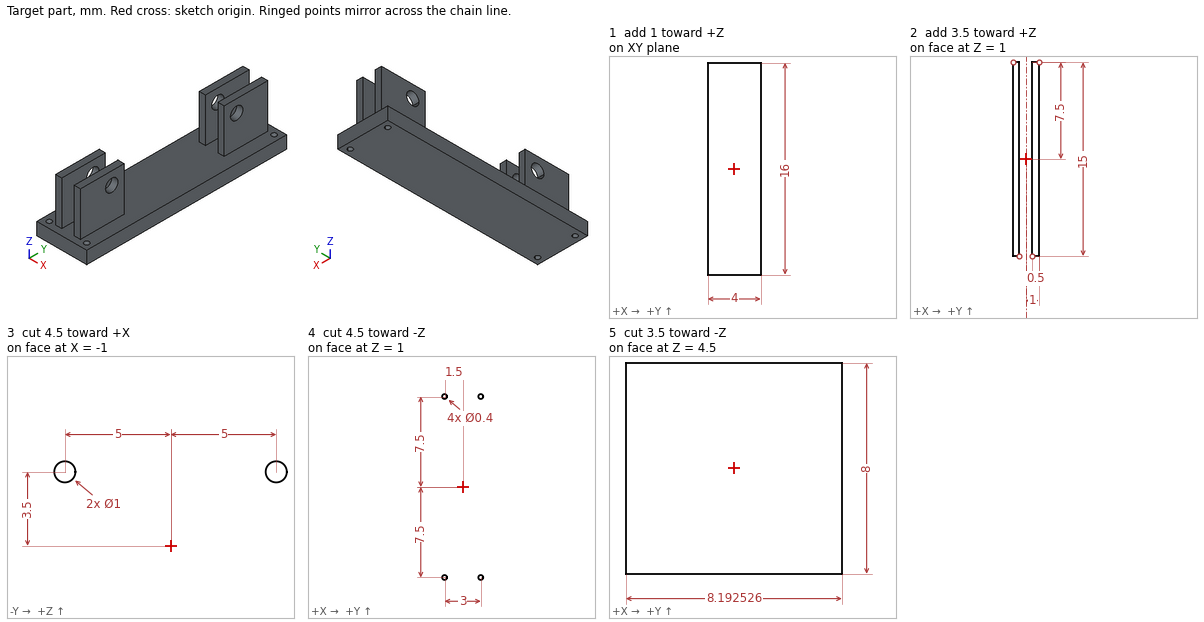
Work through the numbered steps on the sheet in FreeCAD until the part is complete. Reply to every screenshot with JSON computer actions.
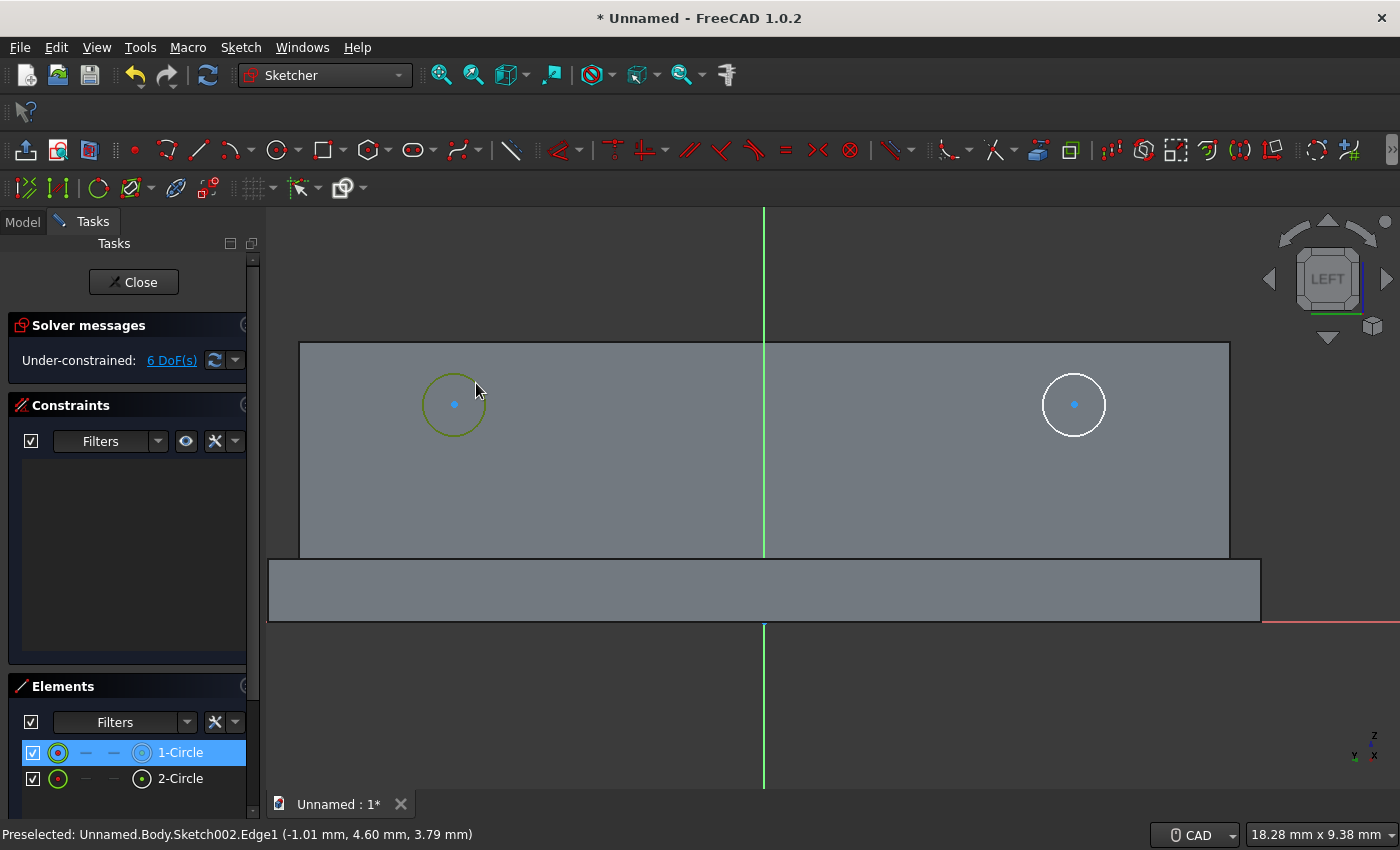
{"action": "left_click", "coordinate": [1096, 383]}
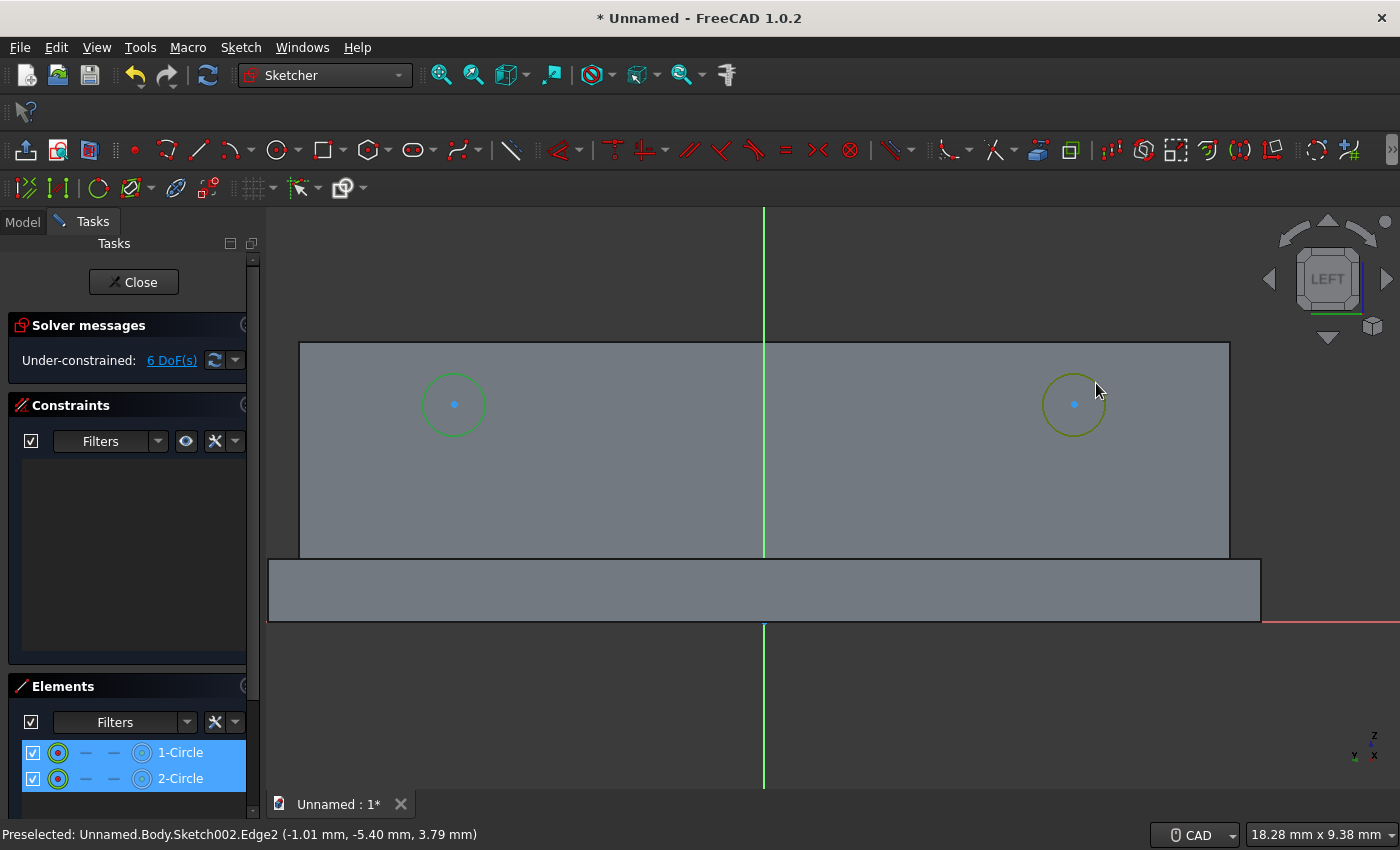
{"action": "key", "text": "e"}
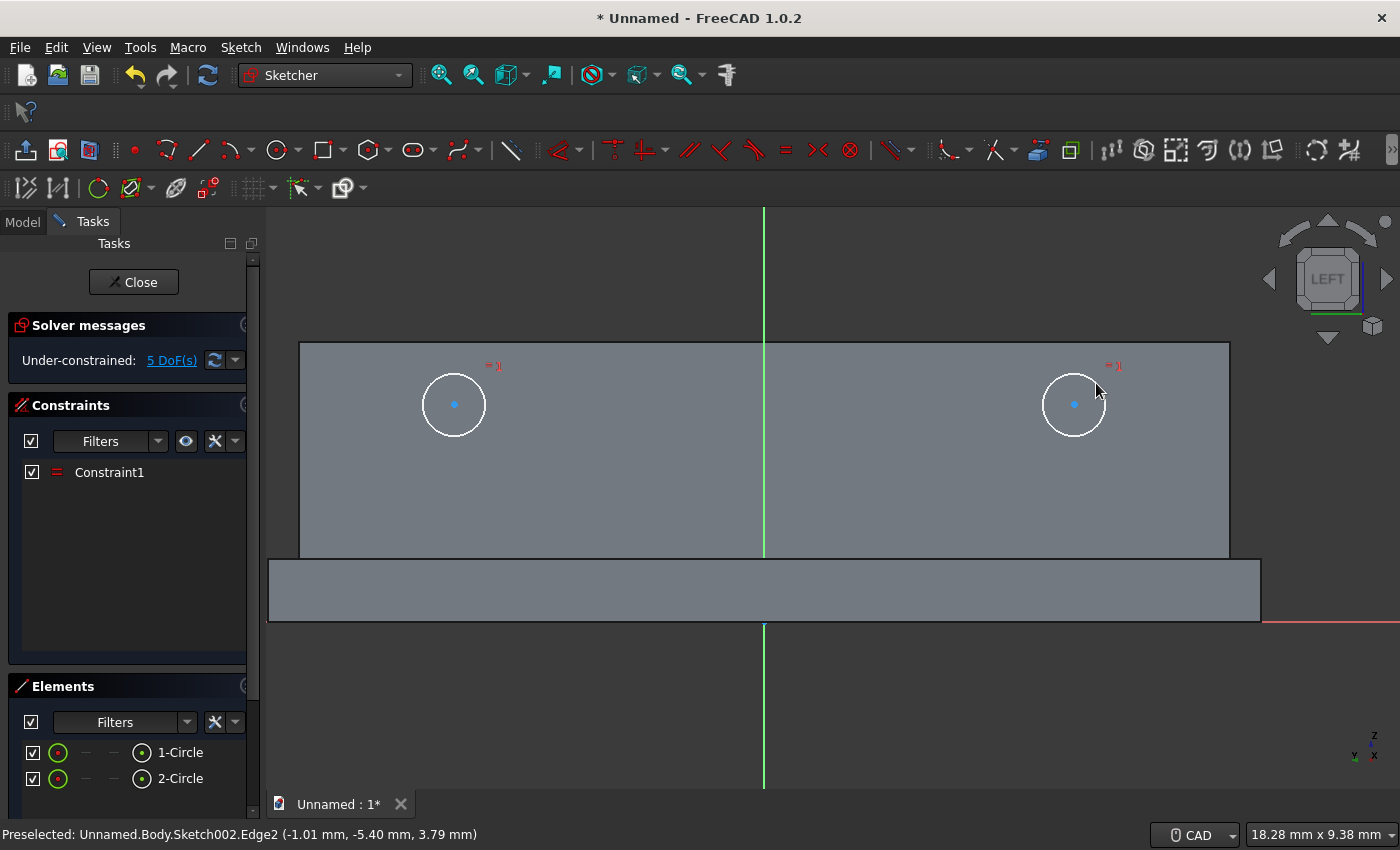
{"action": "left_click", "coordinate": [454, 405]}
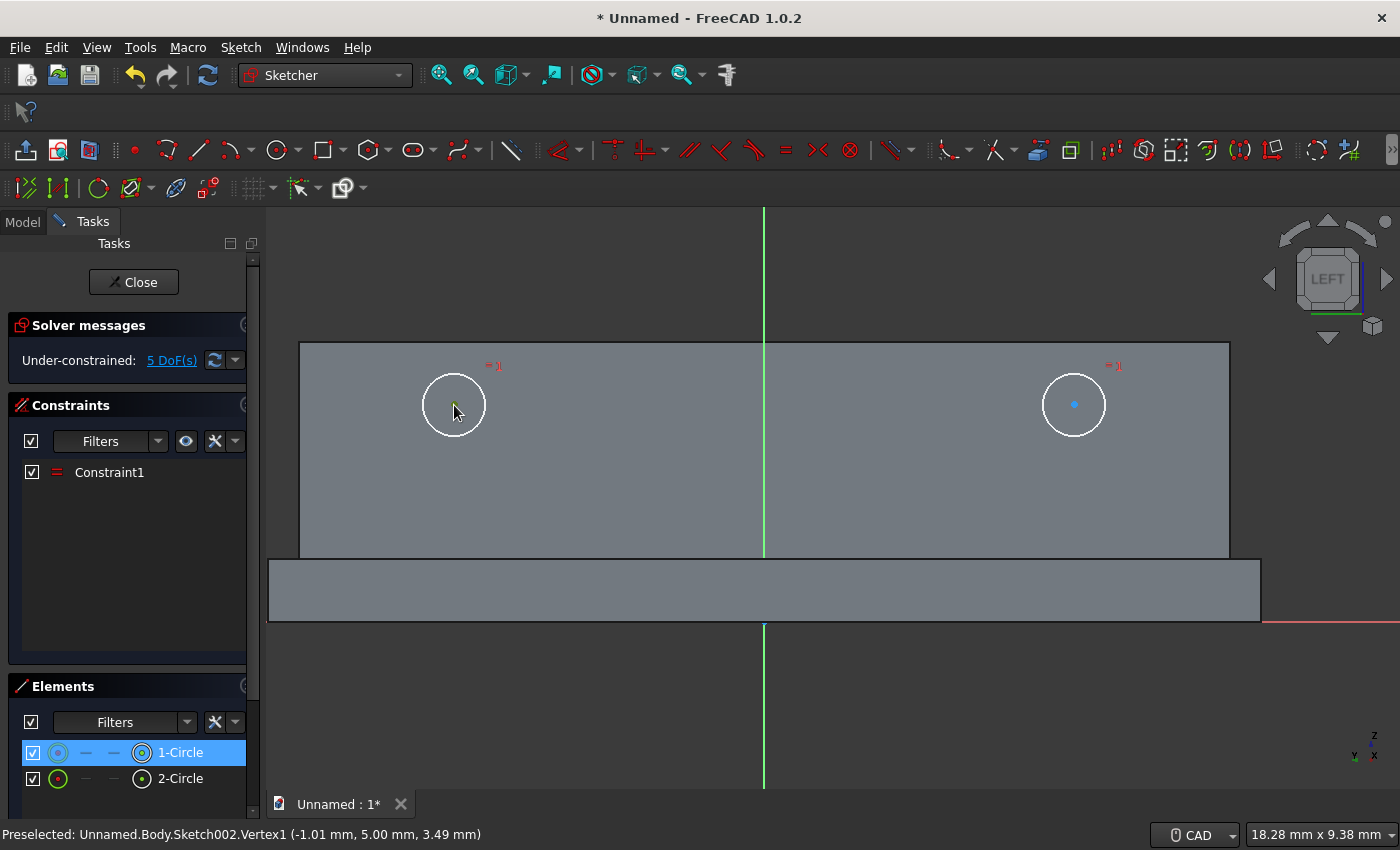
{"action": "left_click", "coordinate": [1074, 405]}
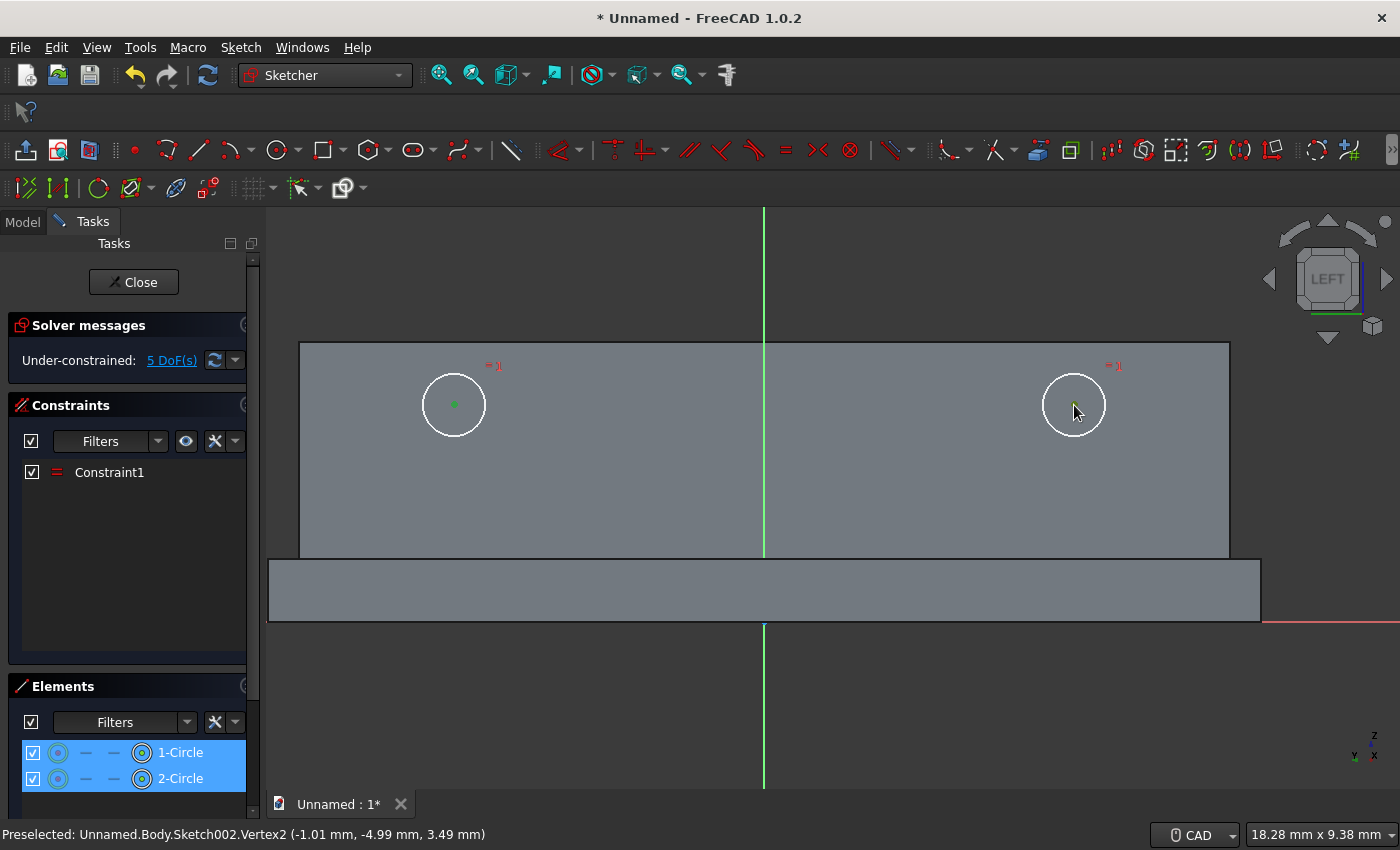
{"action": "key", "text": "h"}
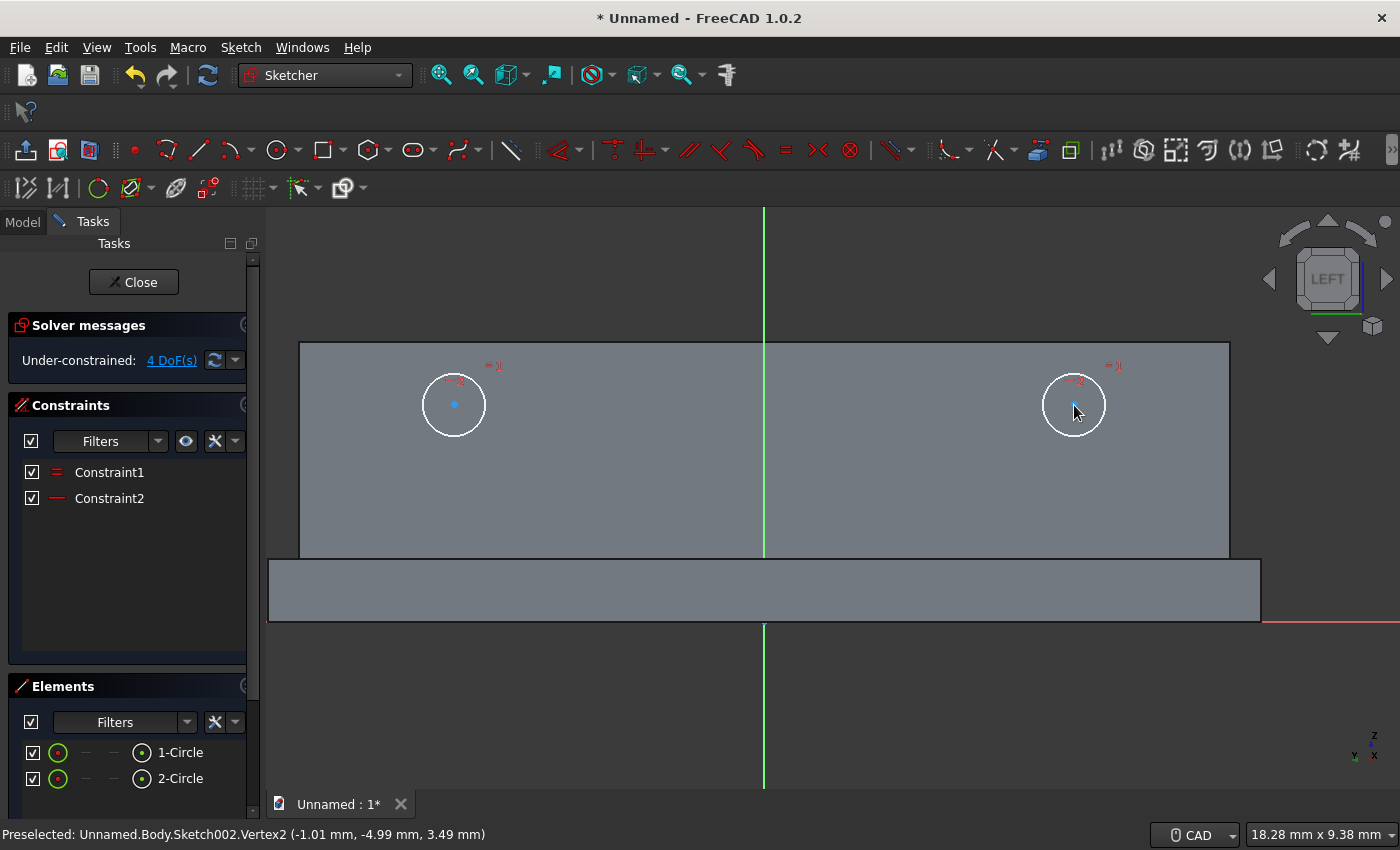
{"action": "key", "text": "d"}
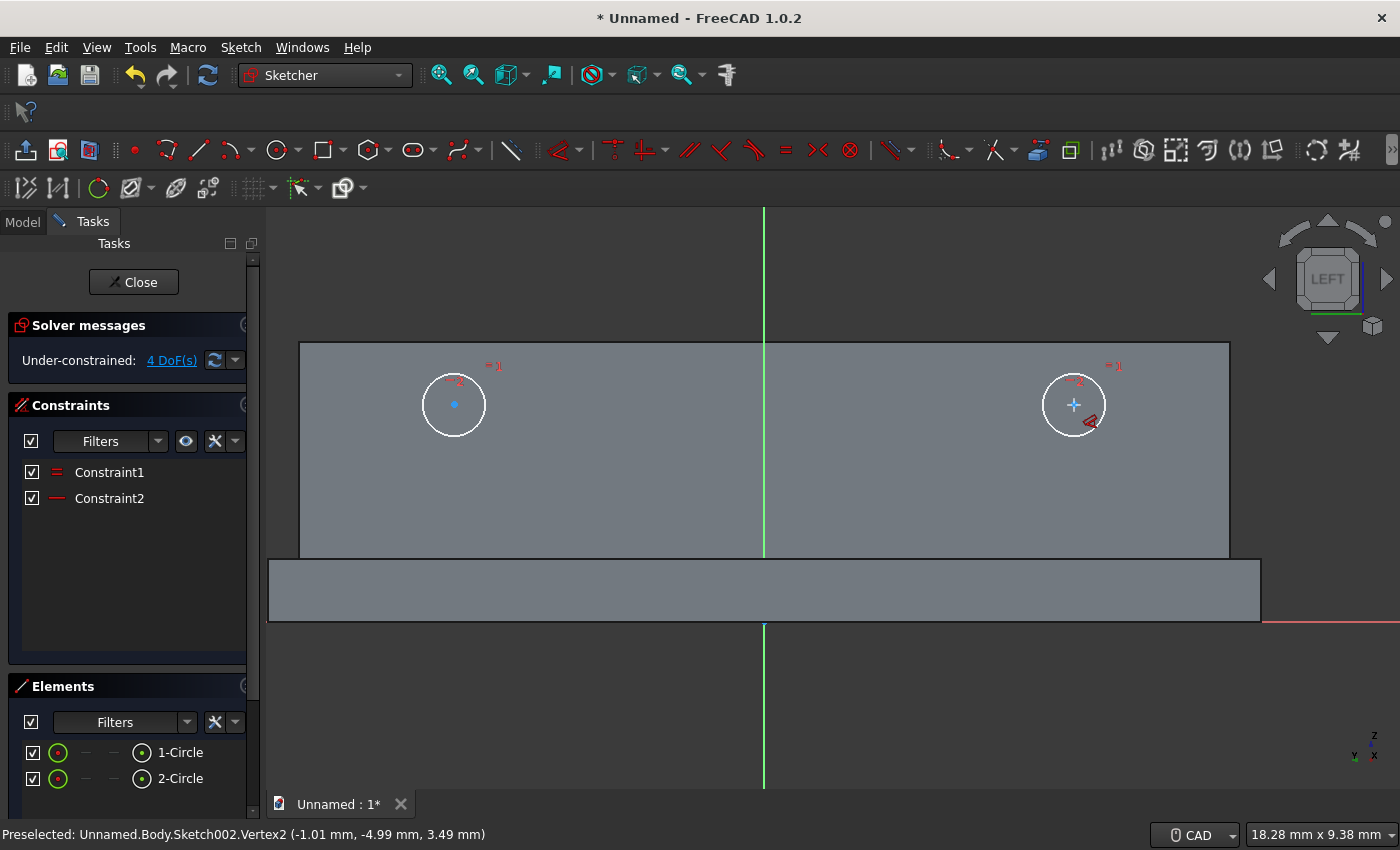
{"action": "left_click", "coordinate": [476, 383]}
{"action": "left_click", "coordinate": [499, 360]}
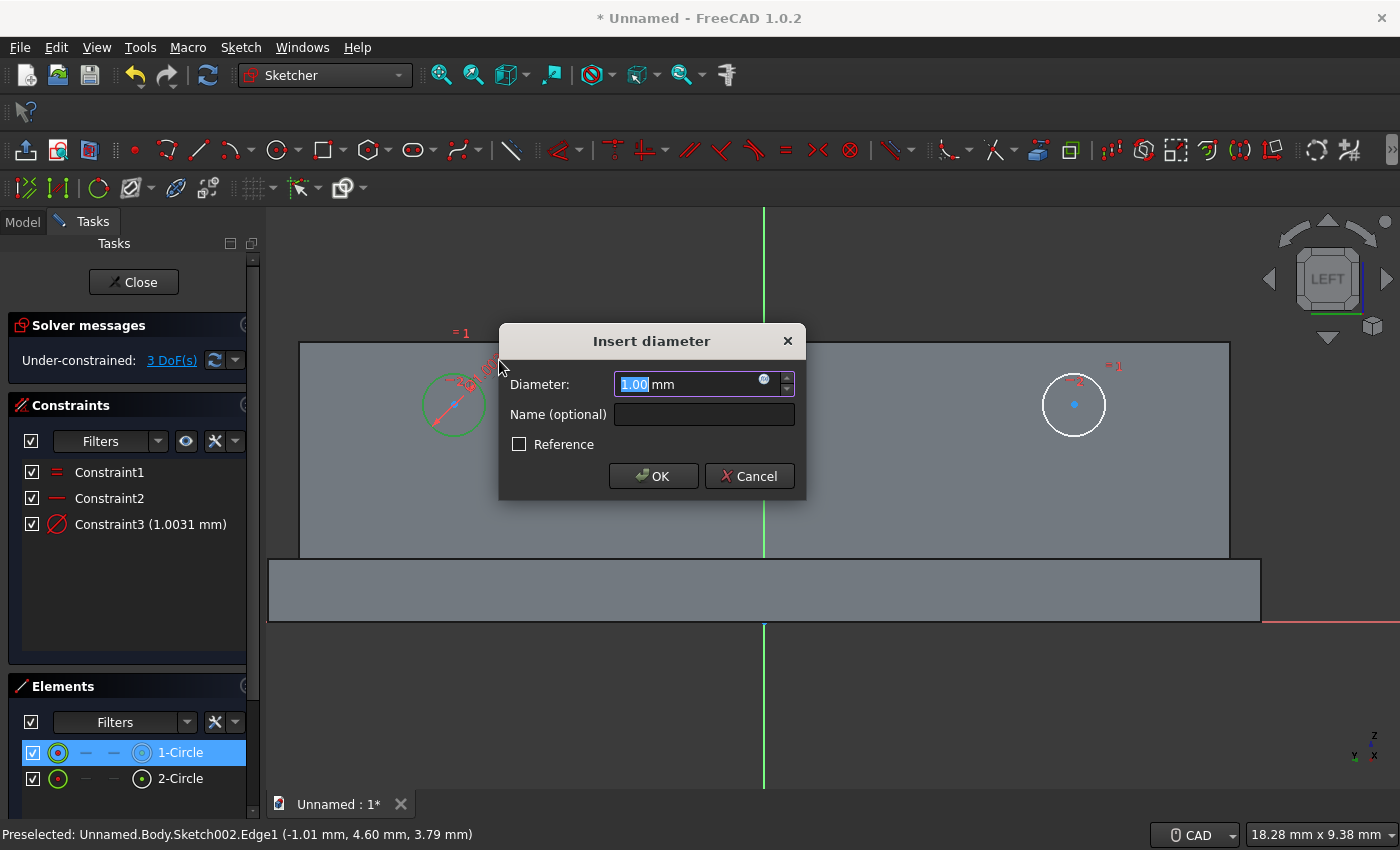
{"action": "type", "text": "1"}
{"action": "key", "text": "Return"}